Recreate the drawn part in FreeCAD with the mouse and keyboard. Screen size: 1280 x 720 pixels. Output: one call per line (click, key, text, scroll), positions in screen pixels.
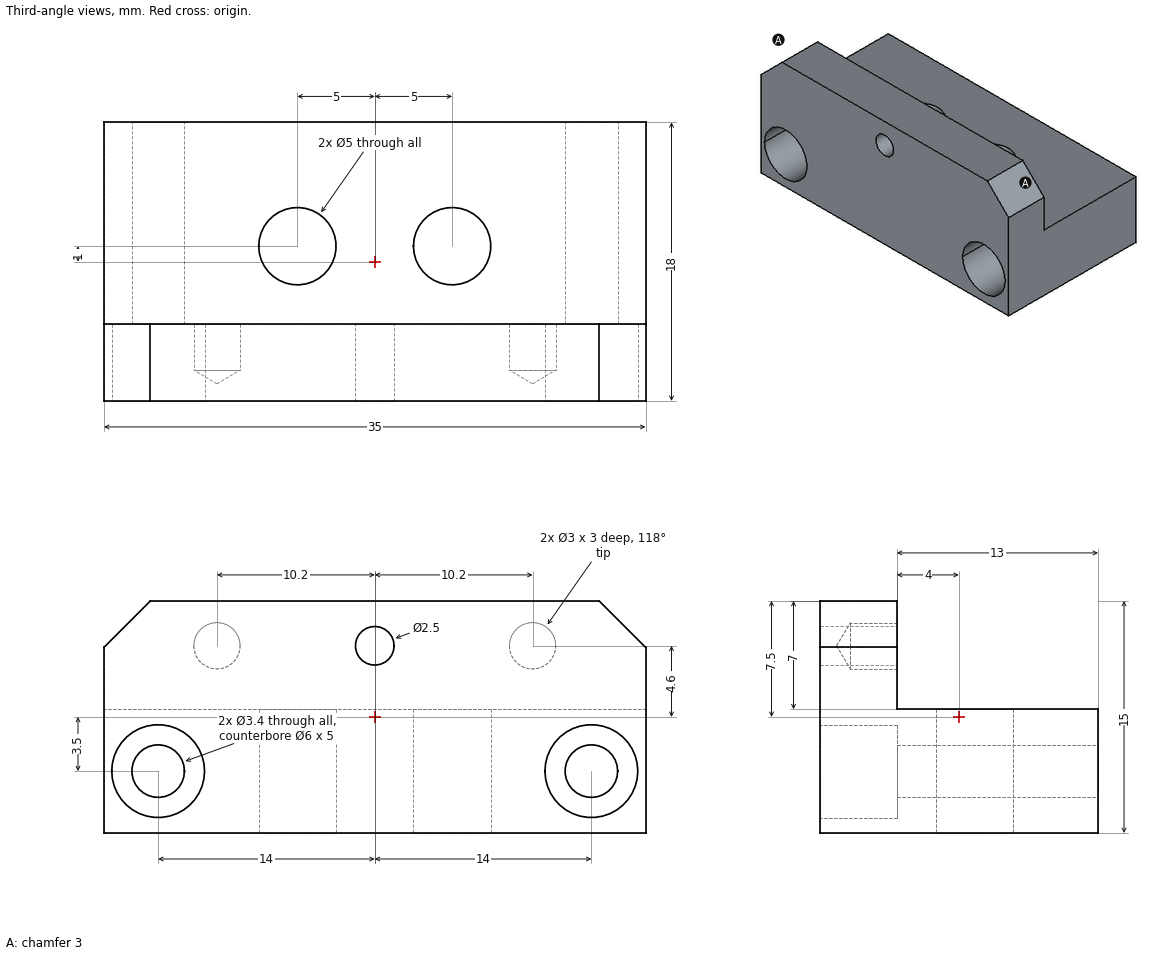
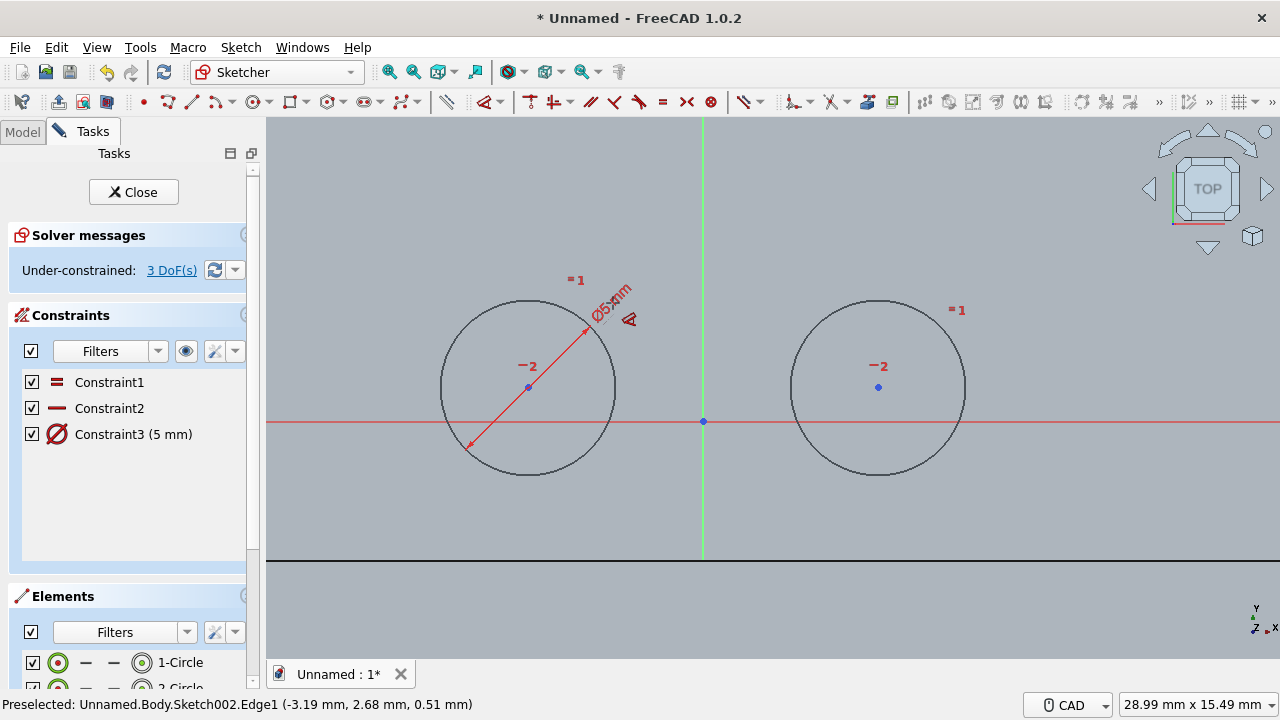
click(528, 388)
click(616, 456)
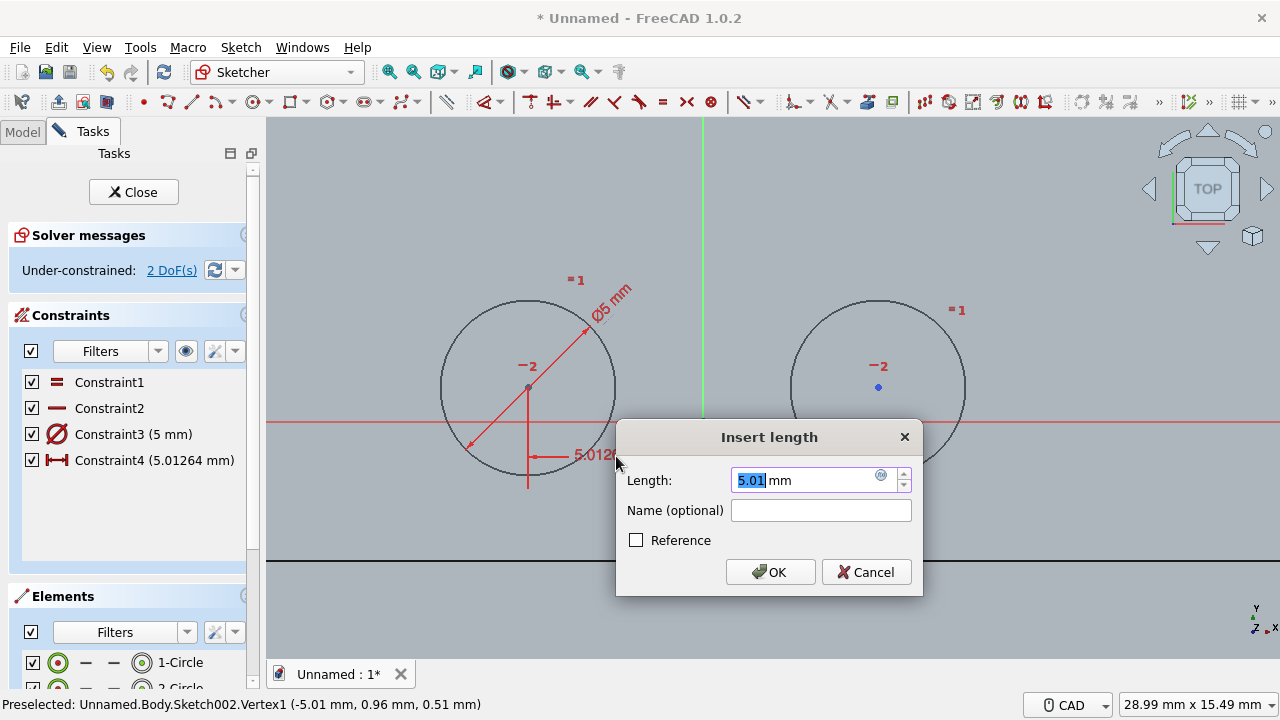
text(5)
key(Return)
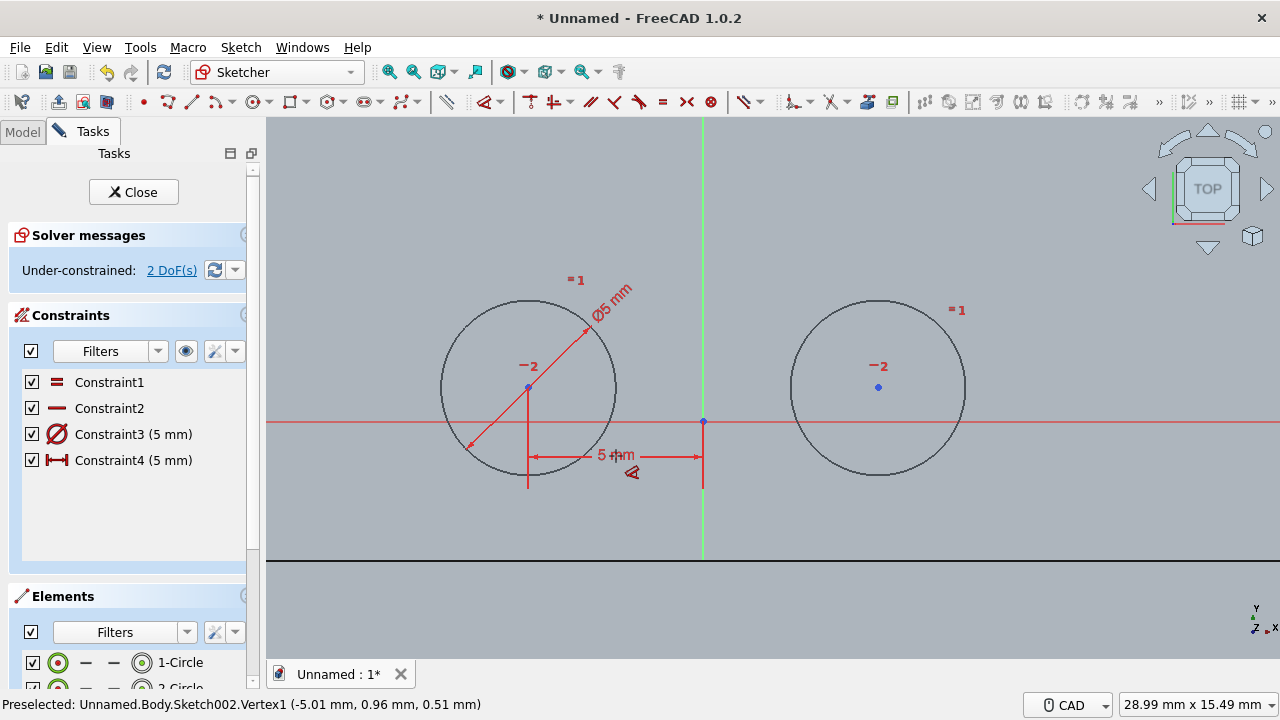
click(528, 388)
click(494, 405)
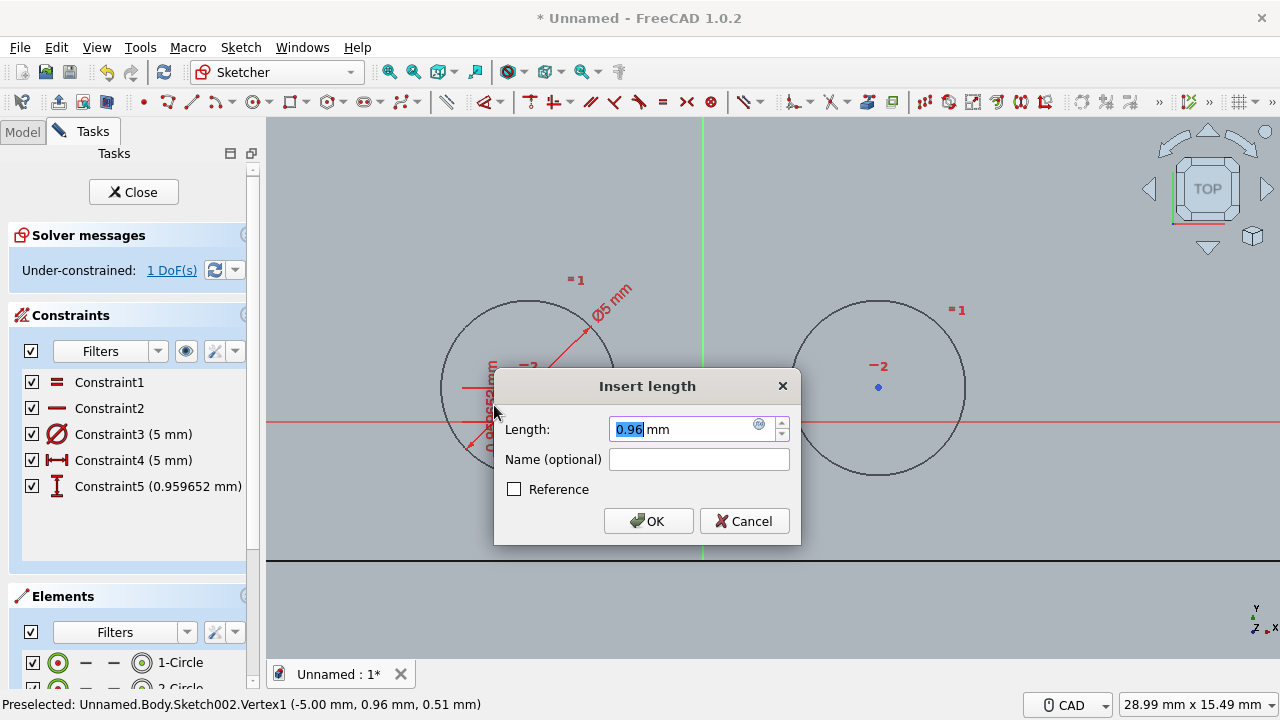
text(1)
key(Return)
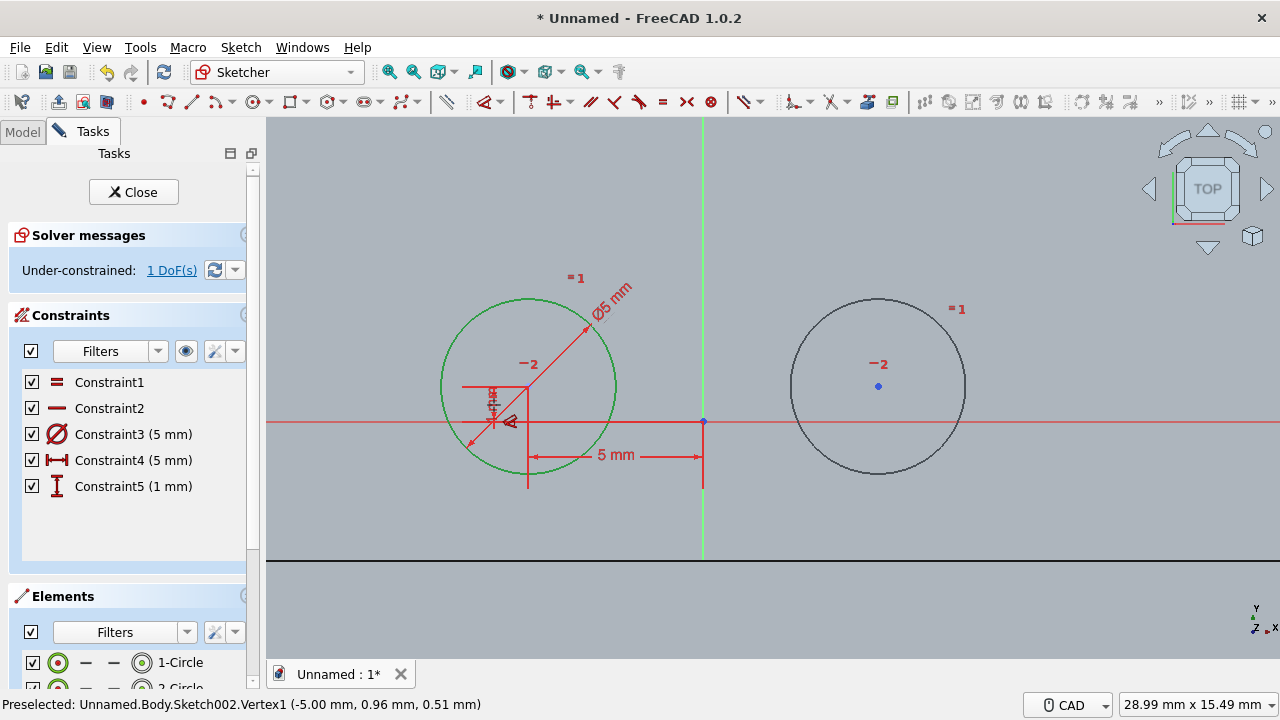
click(878, 387)
click(791, 456)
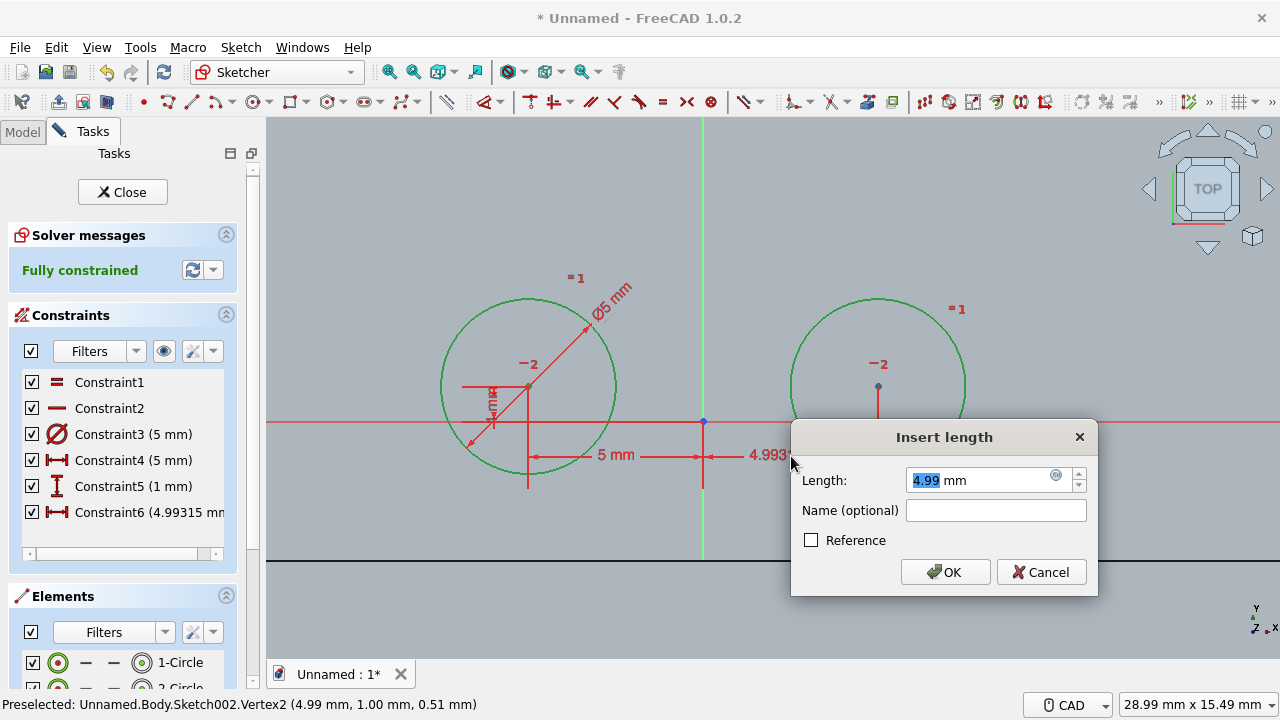
text(5)
key(Return)
key(Escape)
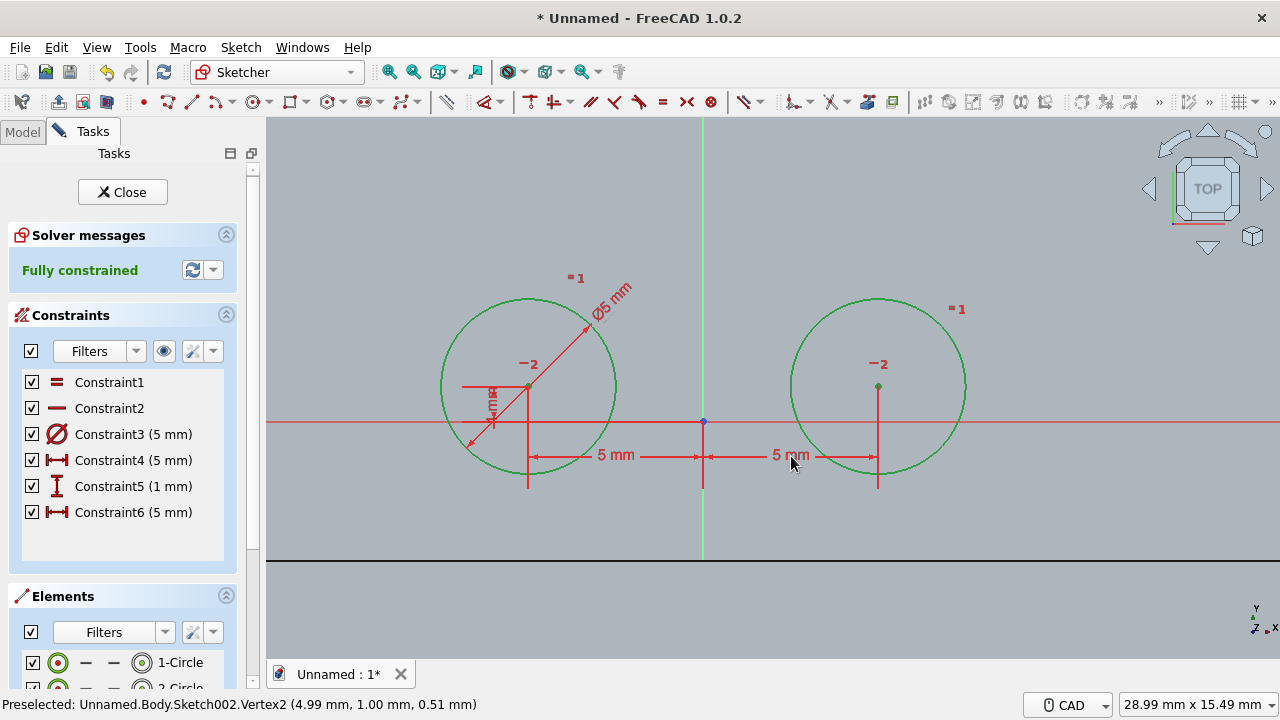
click(123, 192)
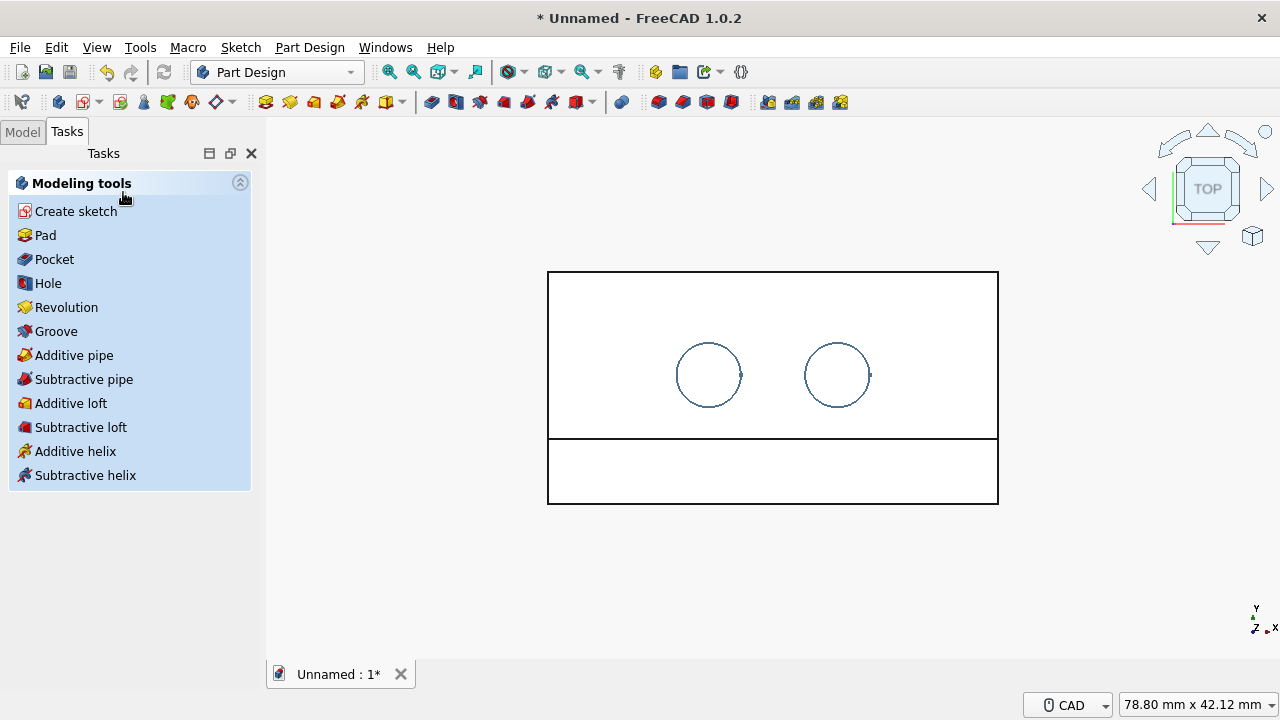
click(456, 102)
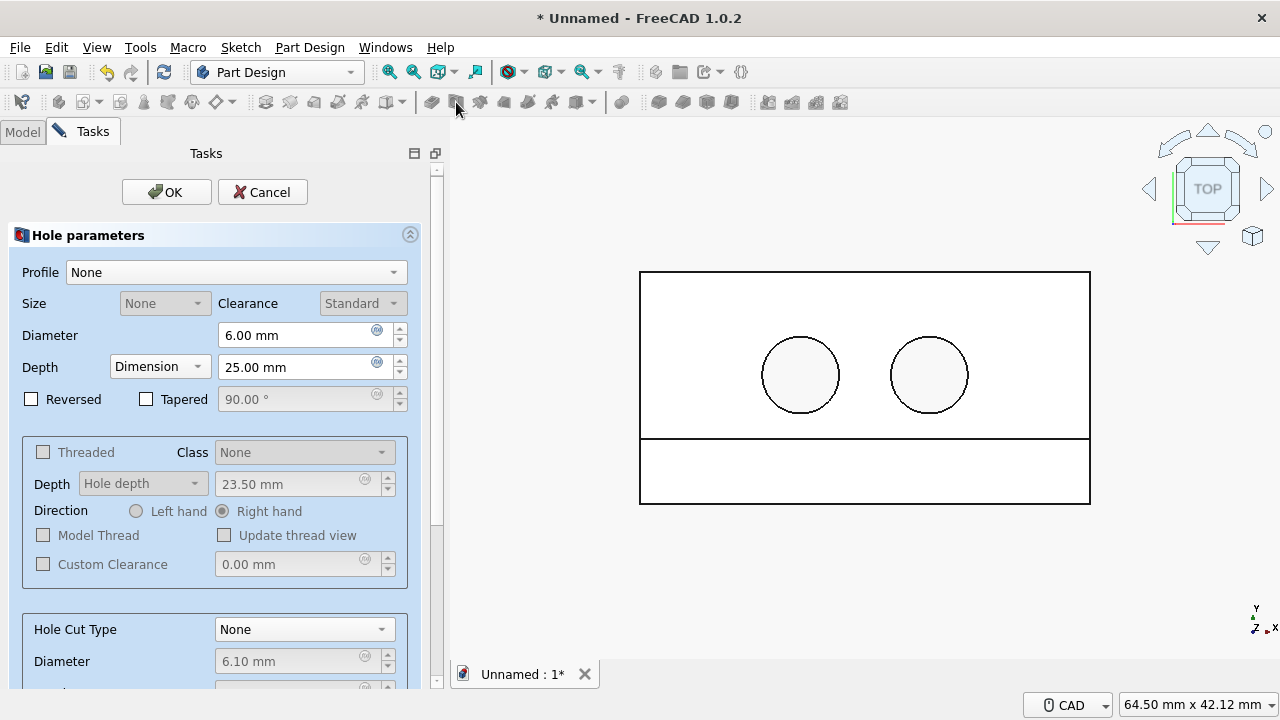
triple_click(305, 335)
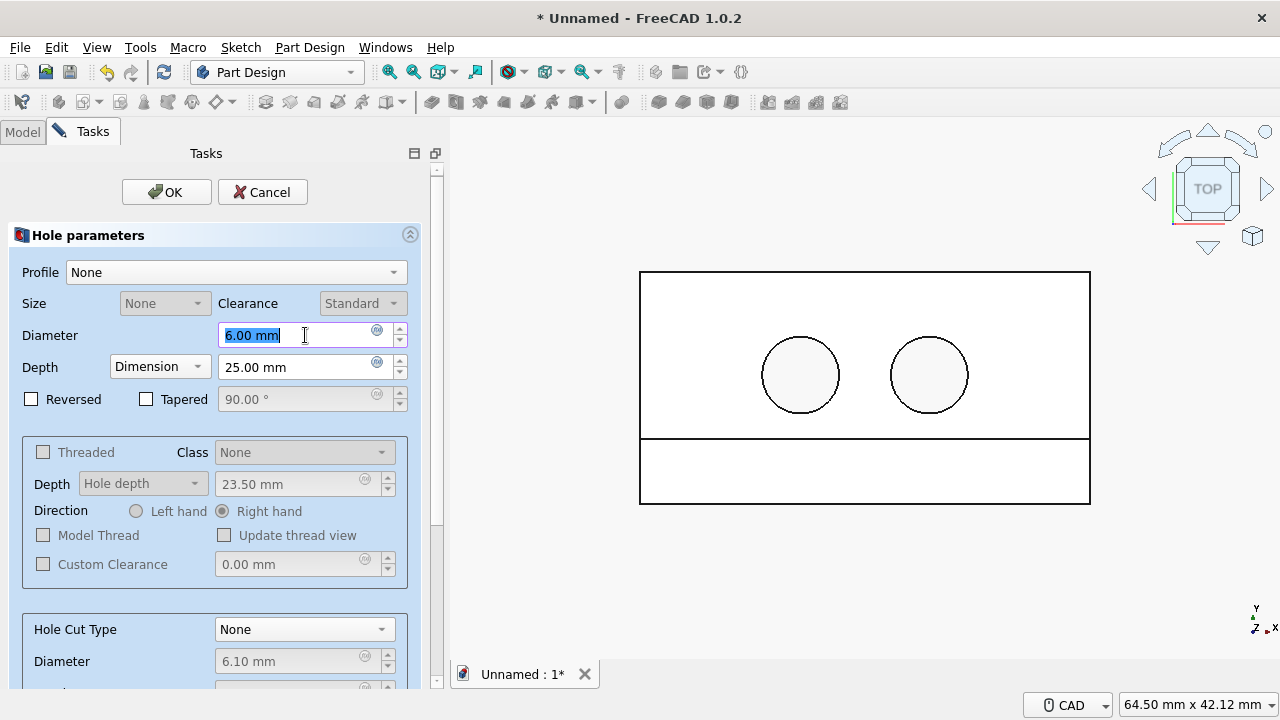
text(5)
key(Tab)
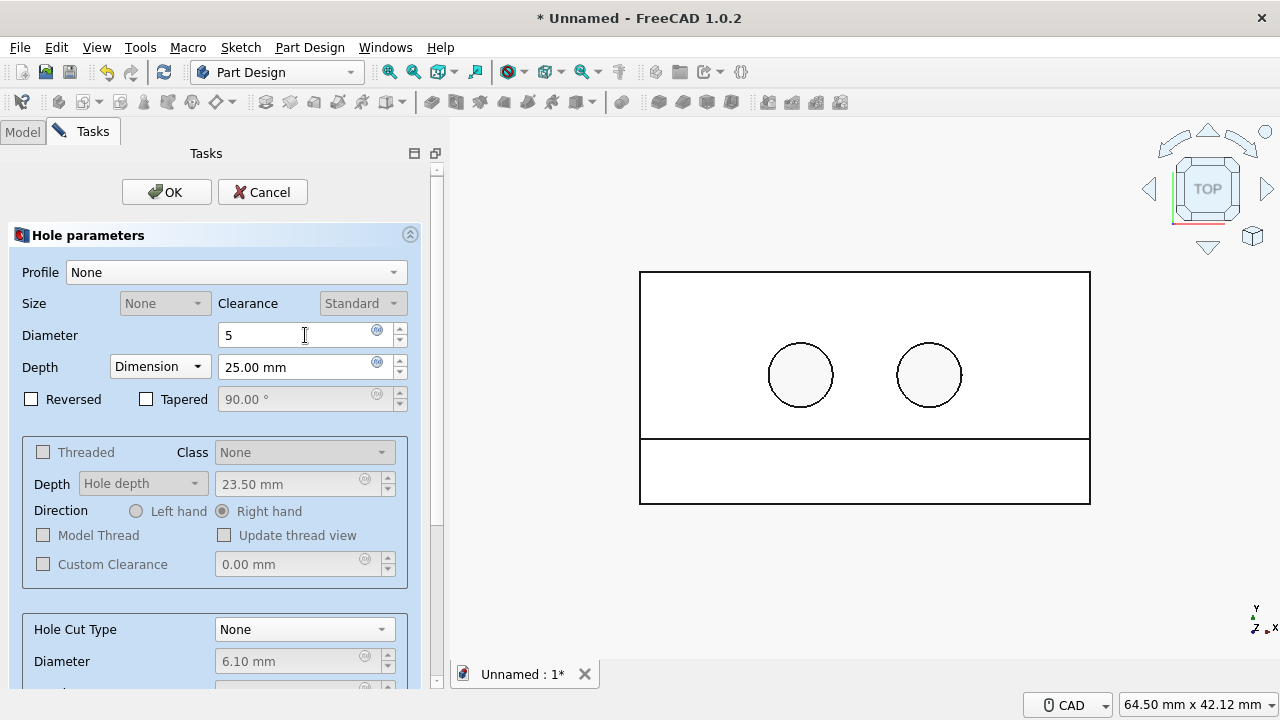
click(161, 366)